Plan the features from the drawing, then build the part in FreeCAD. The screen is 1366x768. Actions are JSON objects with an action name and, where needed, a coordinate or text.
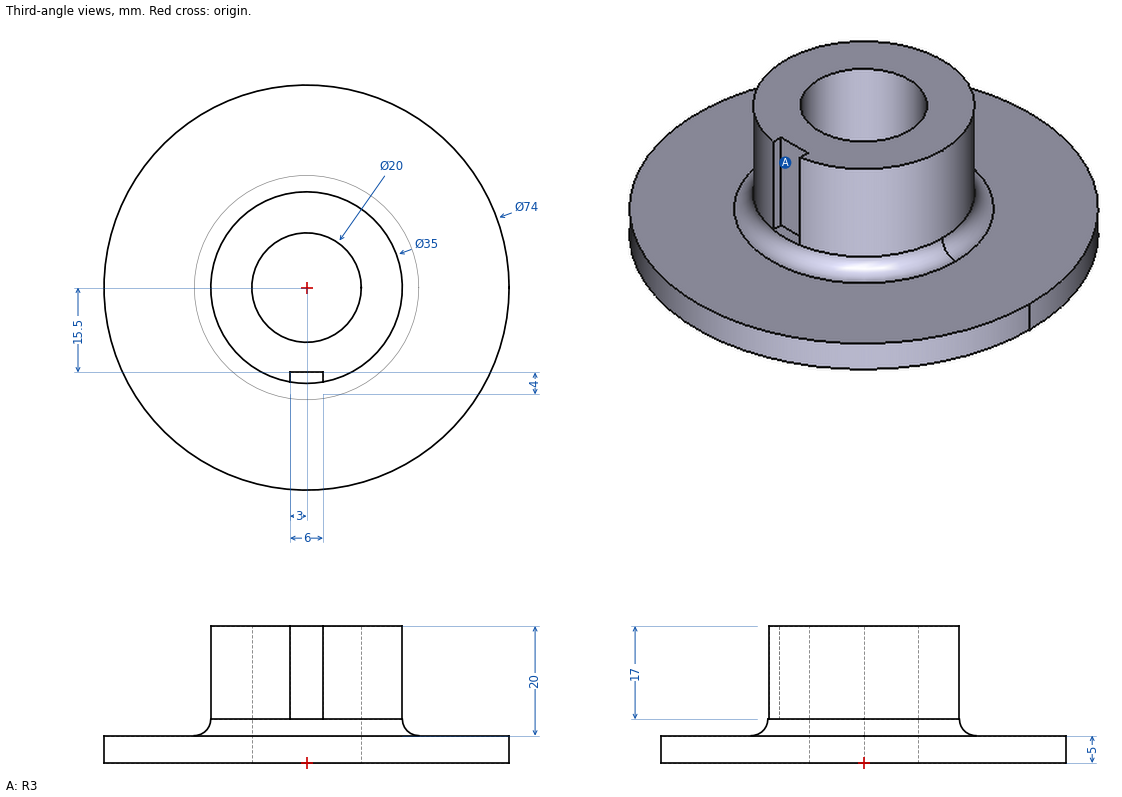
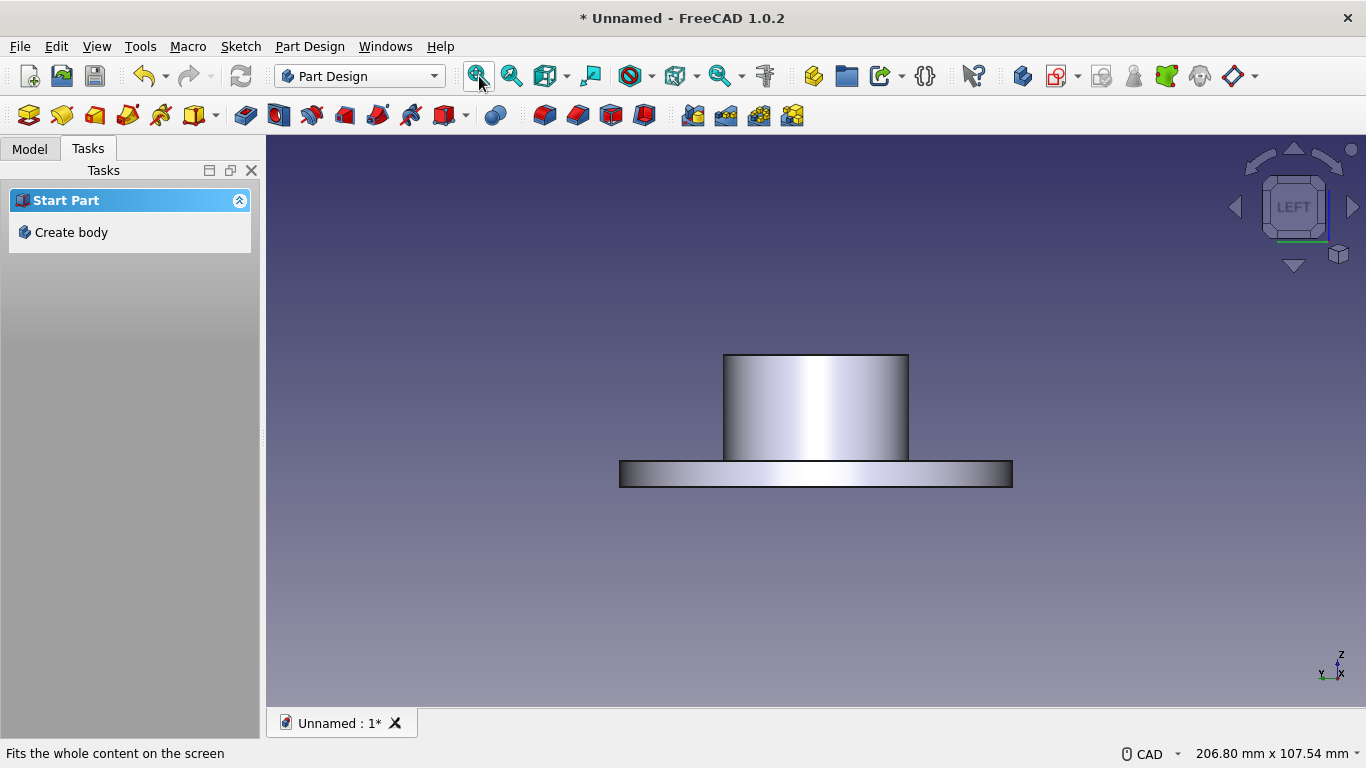
{"action": "key", "text": "v 3"}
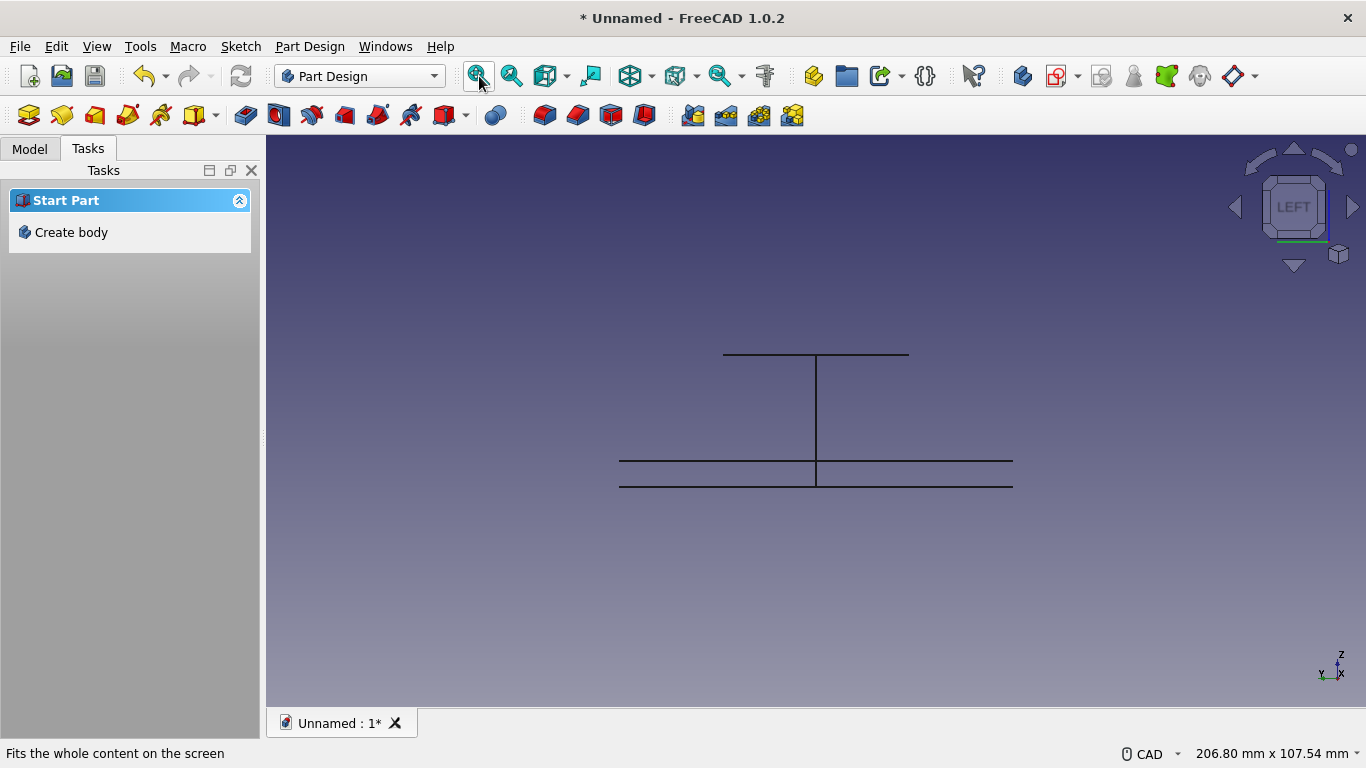
{"action": "key", "text": "0"}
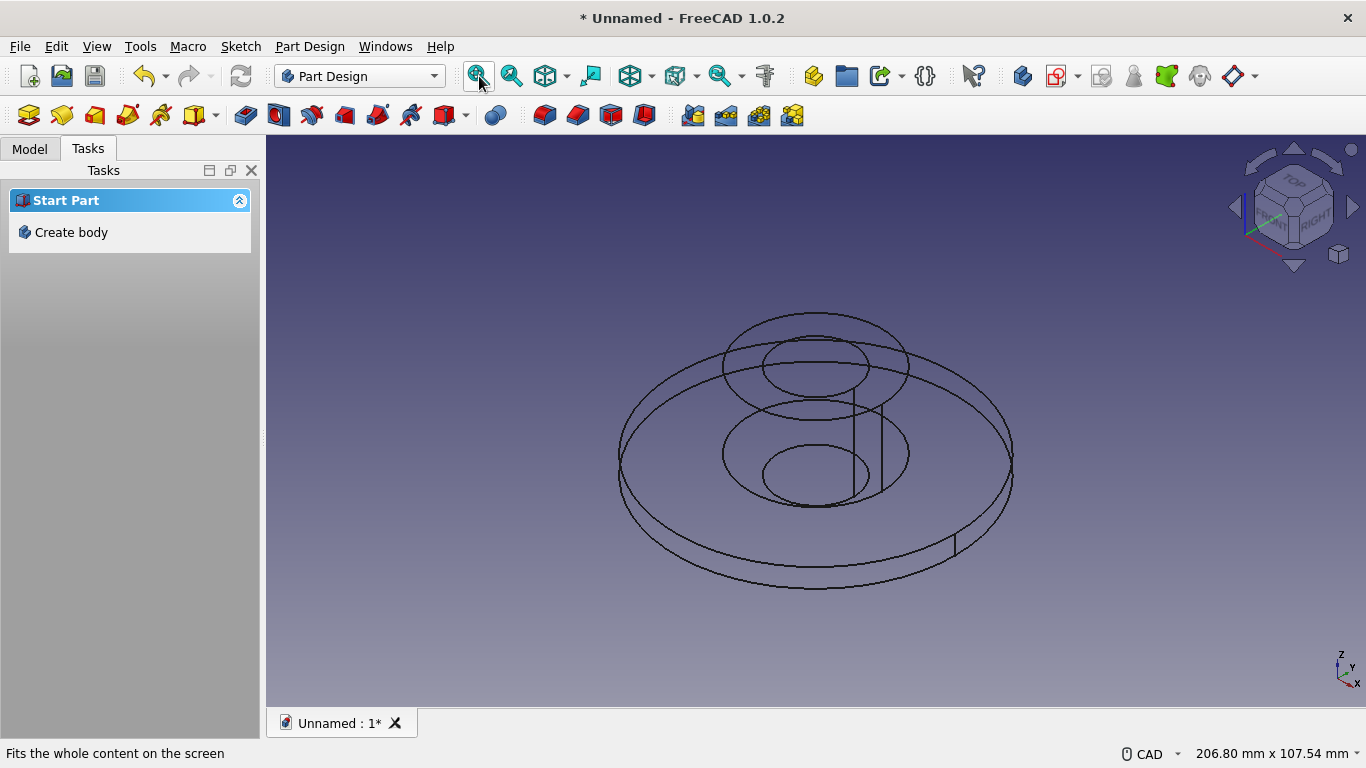
{"action": "left_click", "coordinate": [750, 415]}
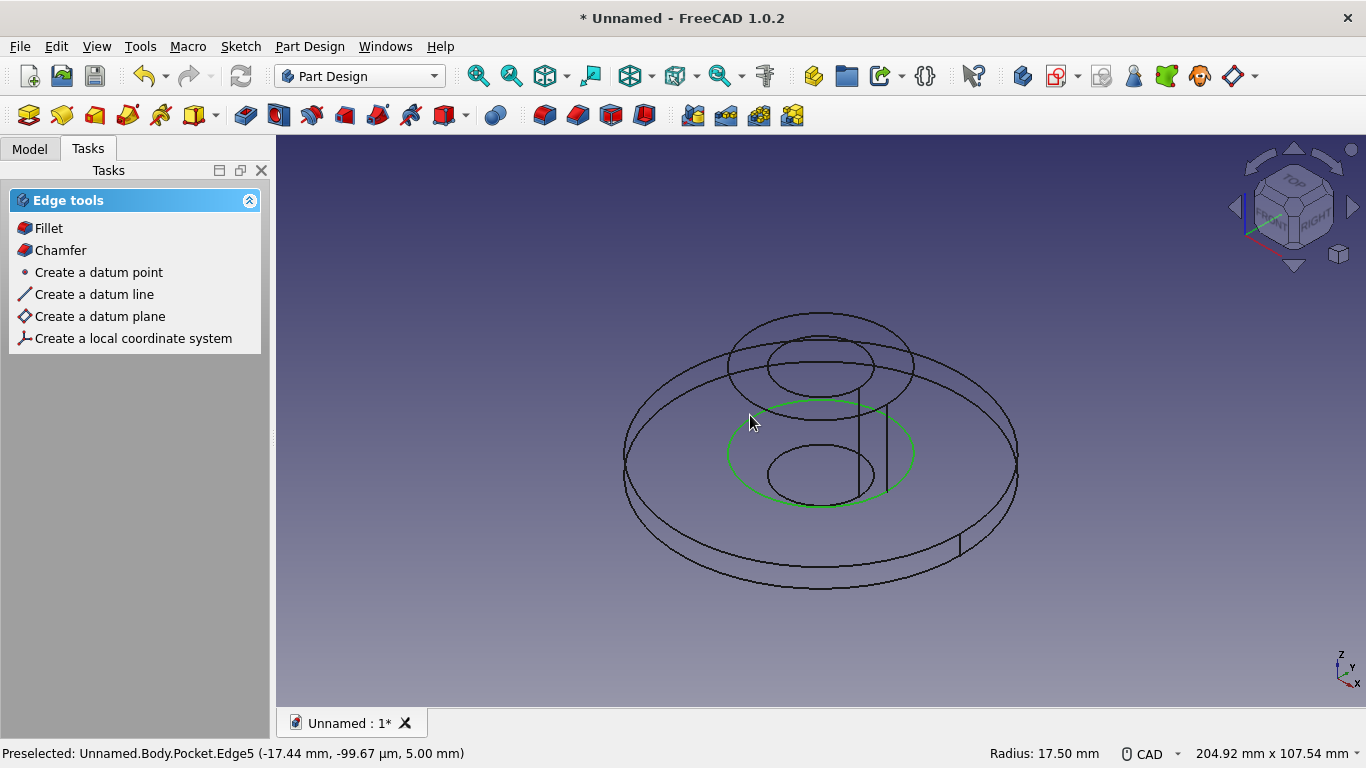
{"action": "key", "text": "v 1"}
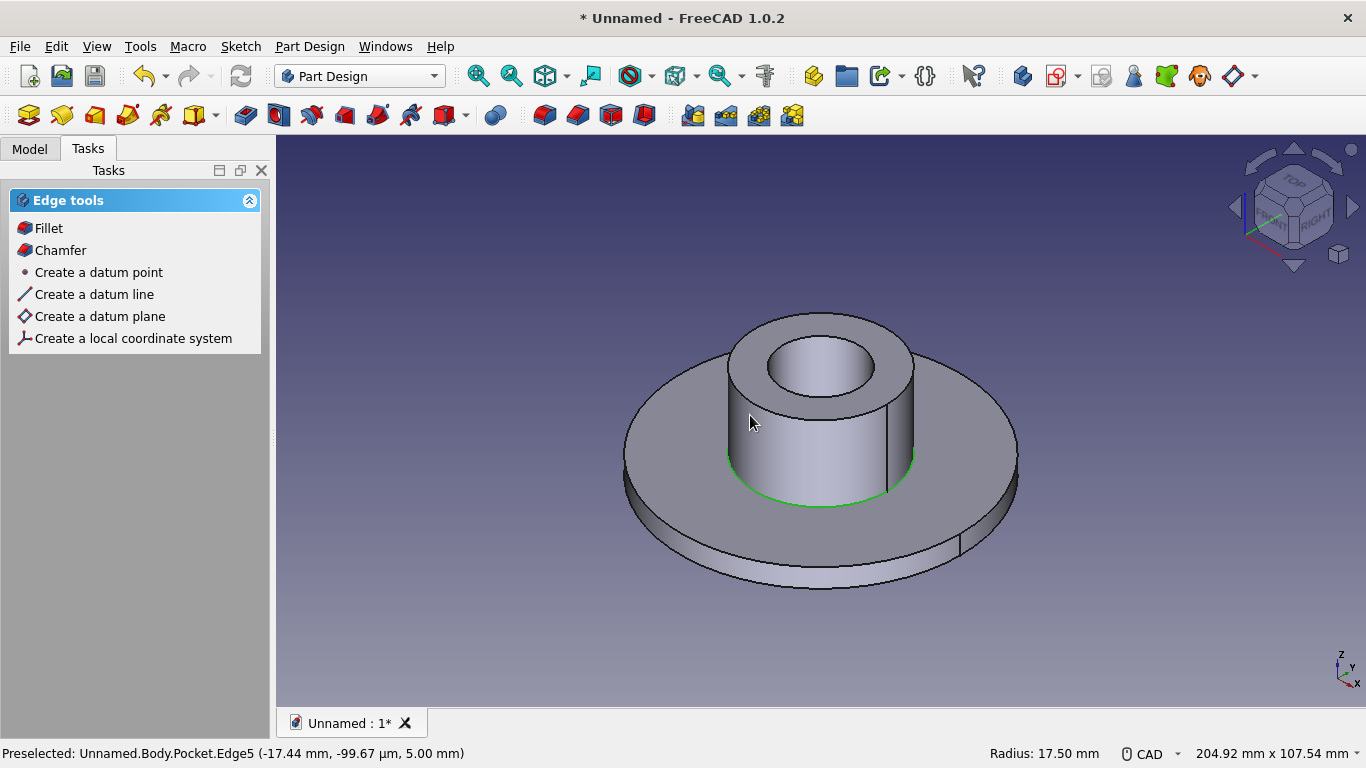
{"action": "left_click", "coordinate": [545, 116]}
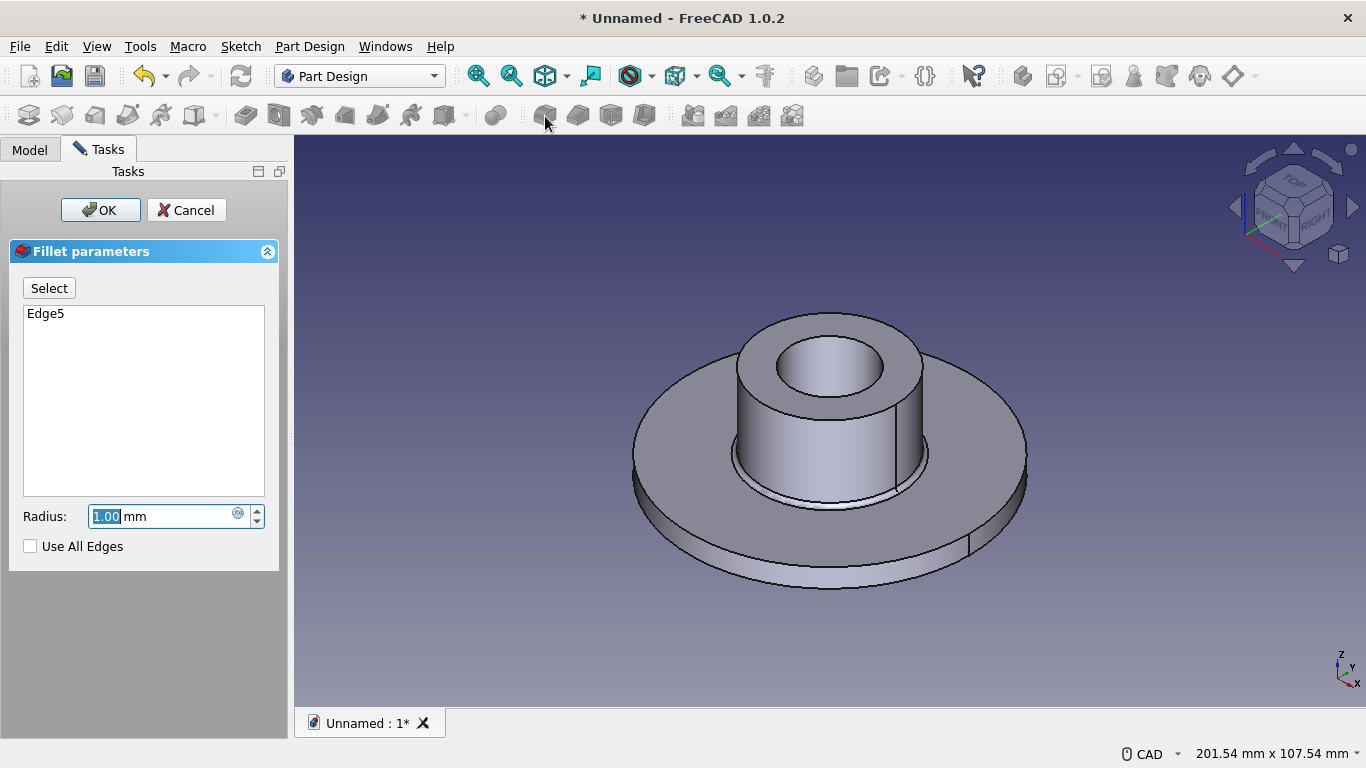
{"action": "type", "text": "3"}
{"action": "key", "text": "Tab"}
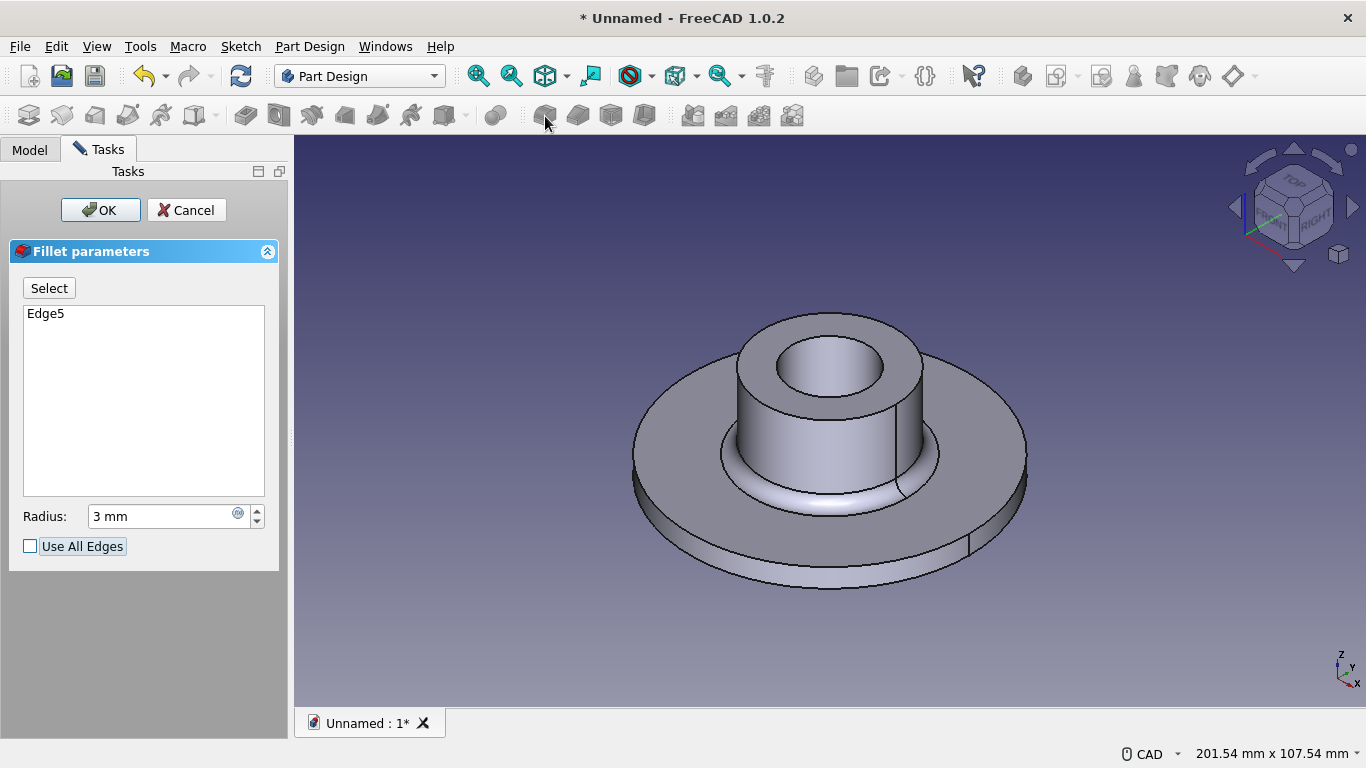
{"action": "left_click", "coordinate": [101, 210]}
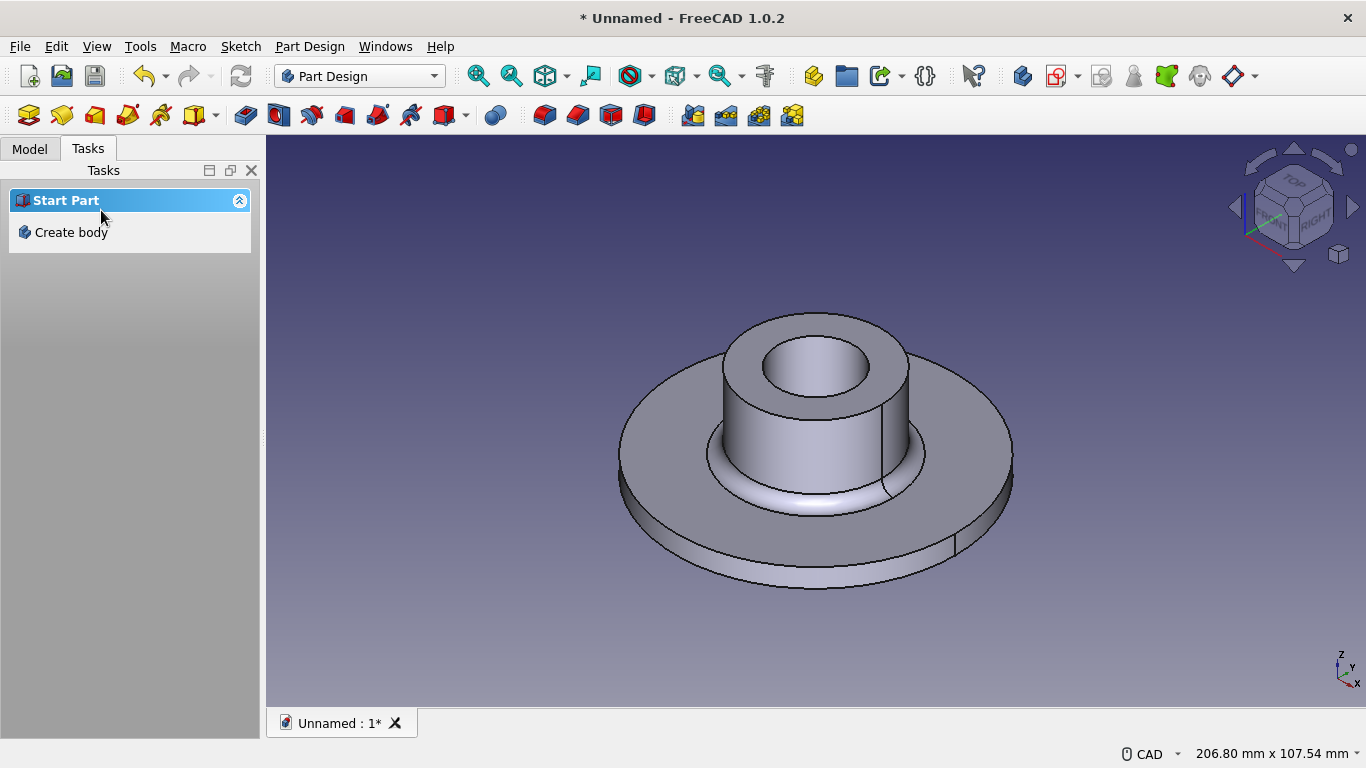
{"action": "left_click", "coordinate": [741, 366]}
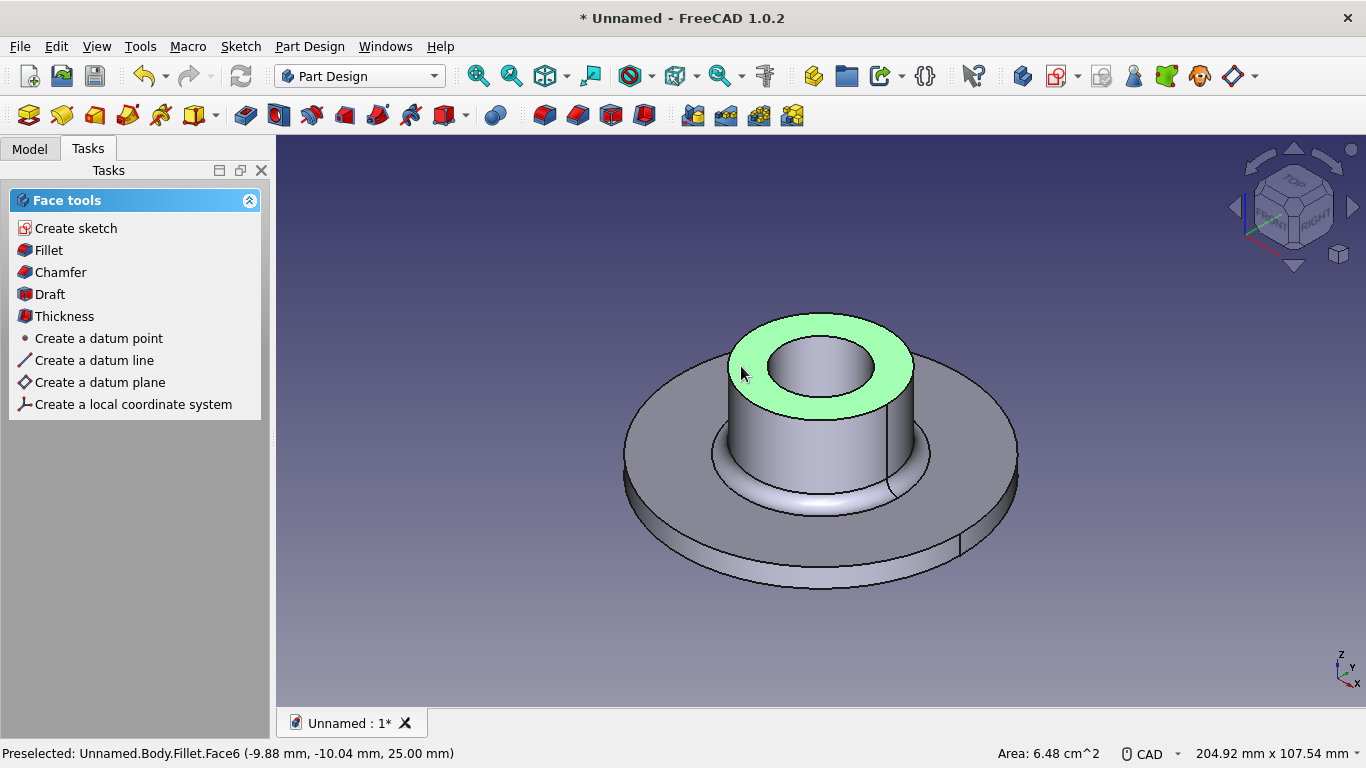
{"action": "left_click", "coordinate": [1056, 76]}